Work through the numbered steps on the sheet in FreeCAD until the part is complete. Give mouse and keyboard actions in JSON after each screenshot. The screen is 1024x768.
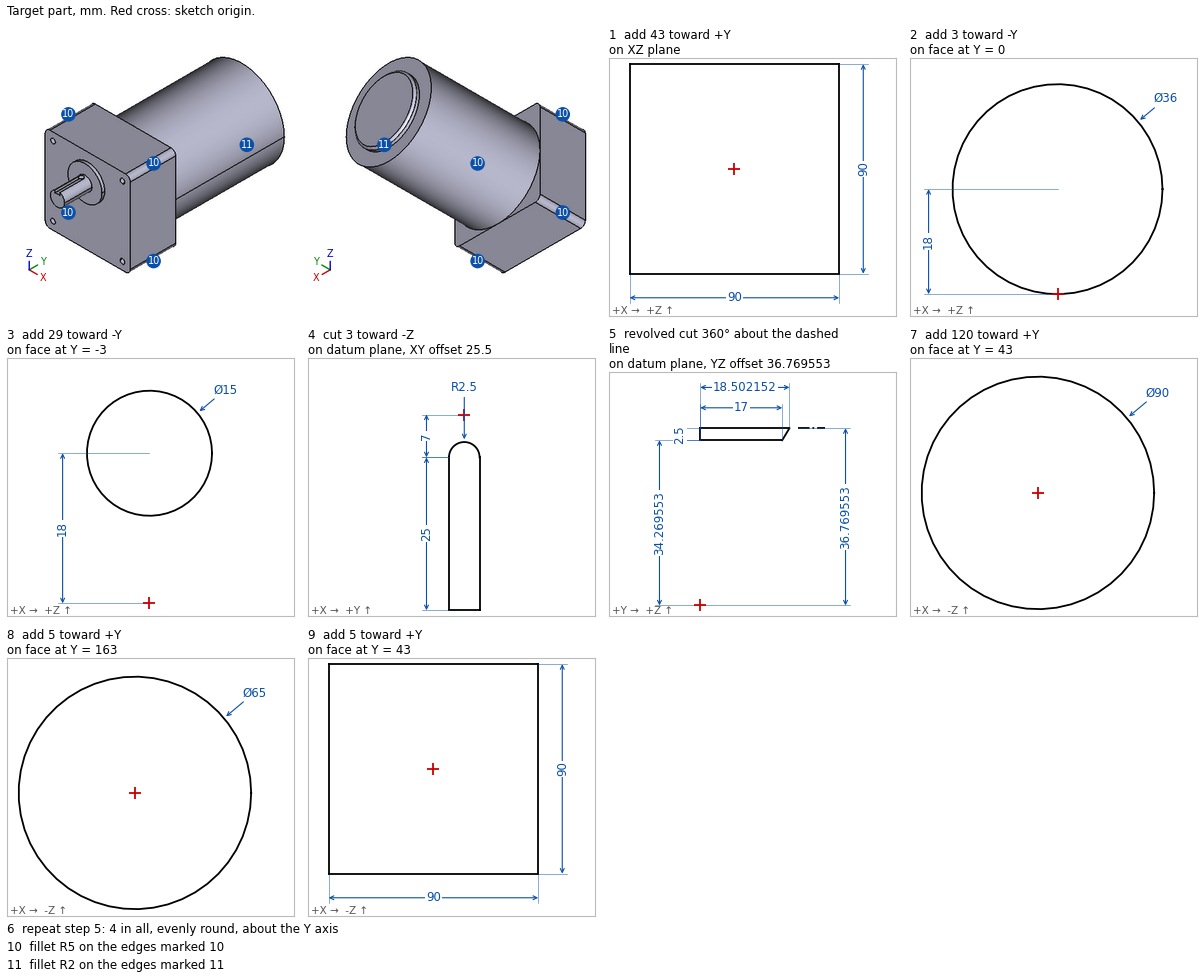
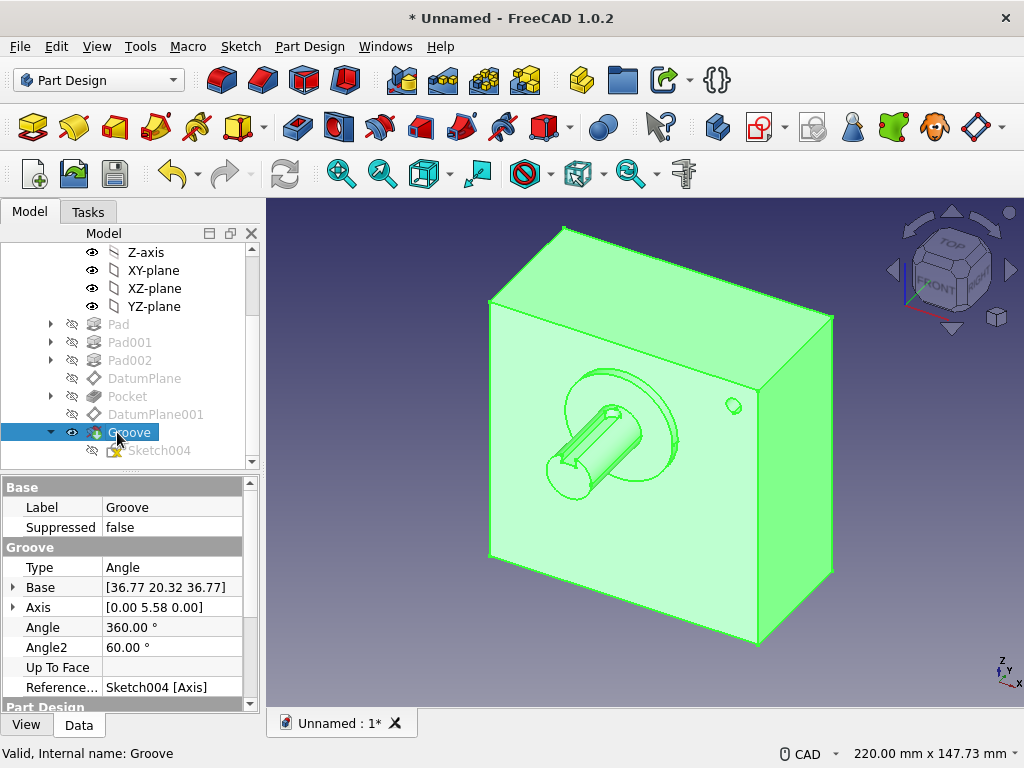
{"action": "left_click", "coordinate": [484, 80]}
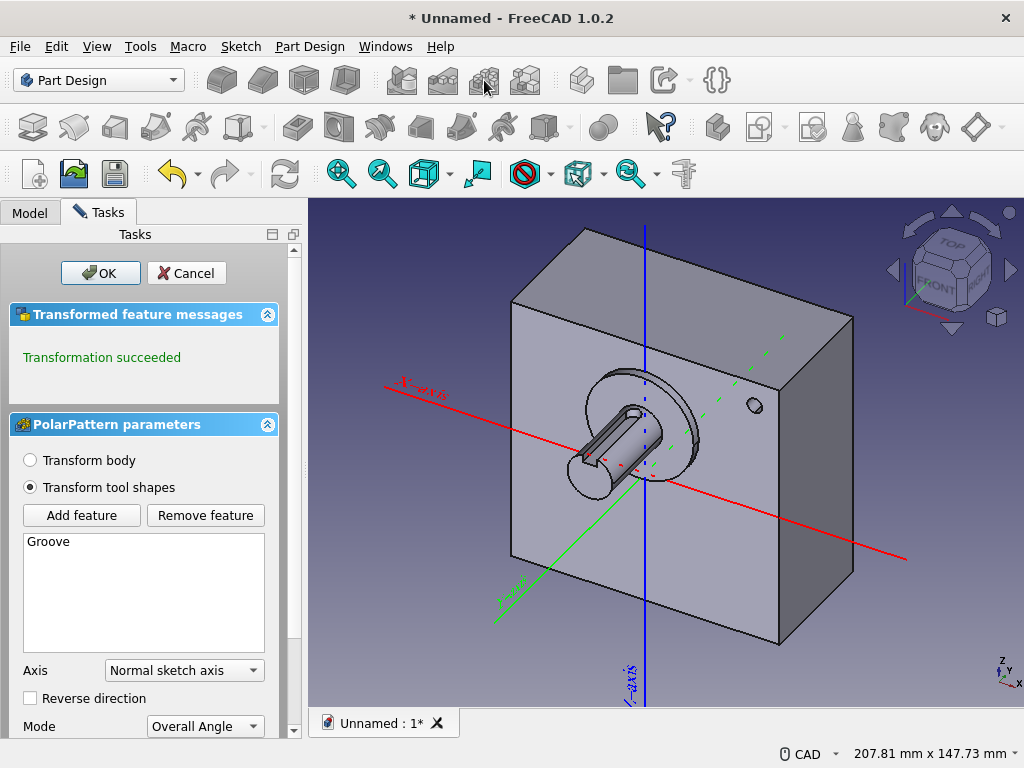
{"action": "left_click", "coordinate": [185, 670]}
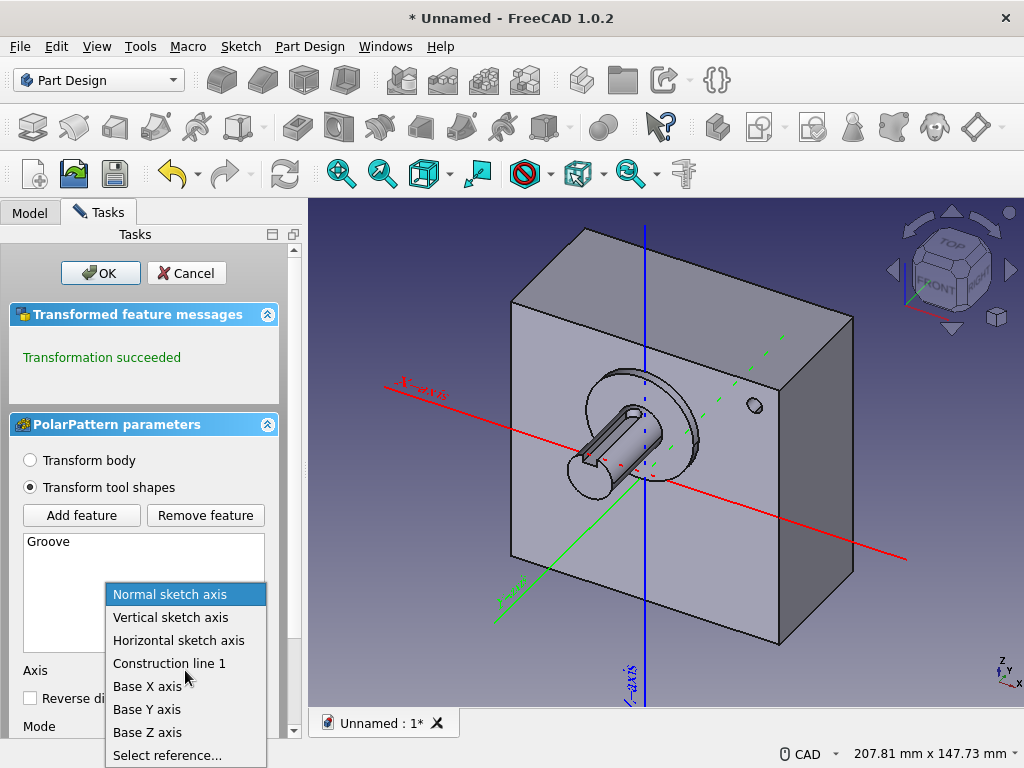
{"action": "left_click", "coordinate": [184, 710]}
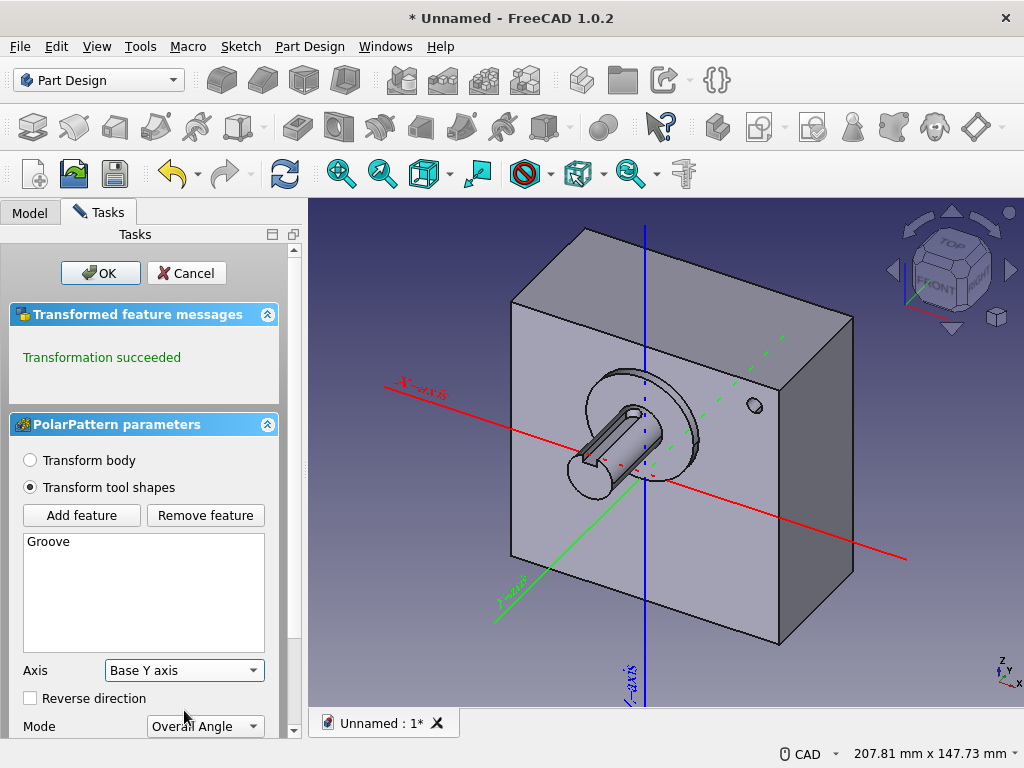
{"action": "scroll", "coordinate": [294, 491], "scroll_direction": "down", "scroll_amount": 3}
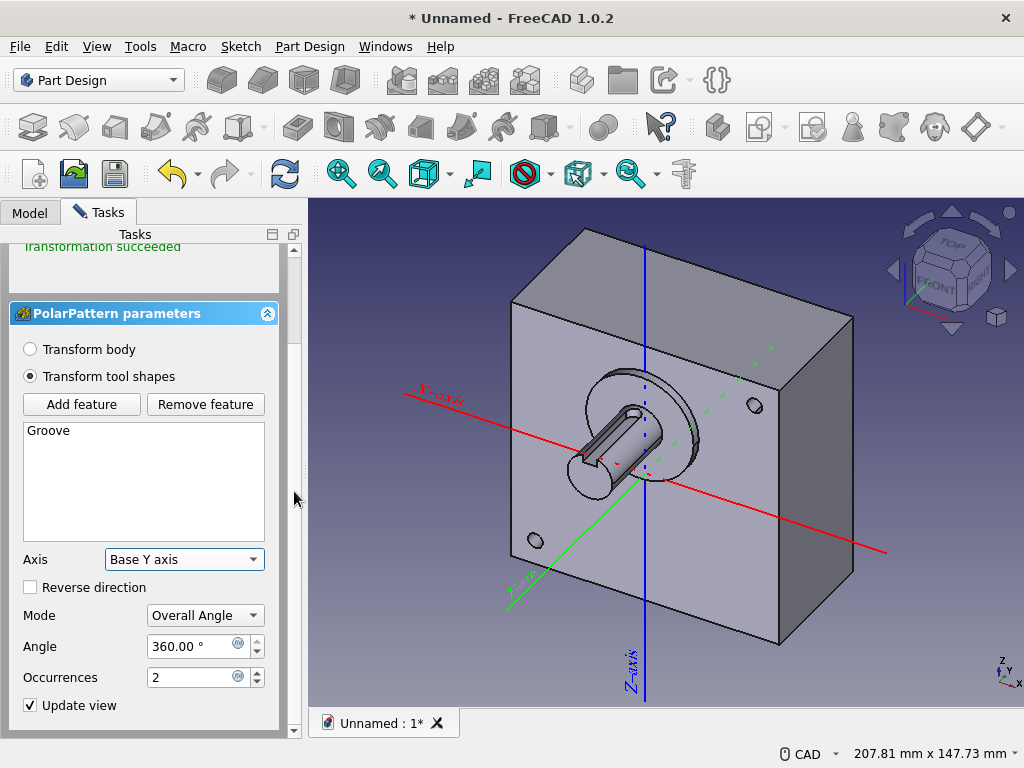
{"action": "triple_click", "coordinate": [199, 678]}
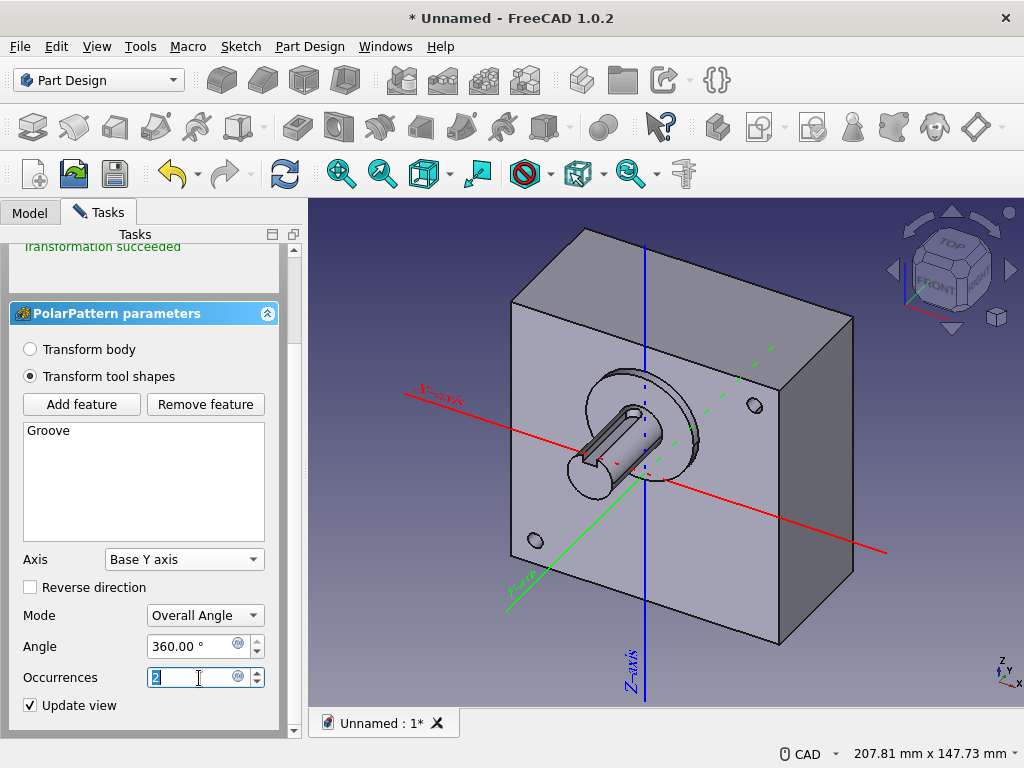
{"action": "type", "text": "4"}
{"action": "key", "text": "Tab"}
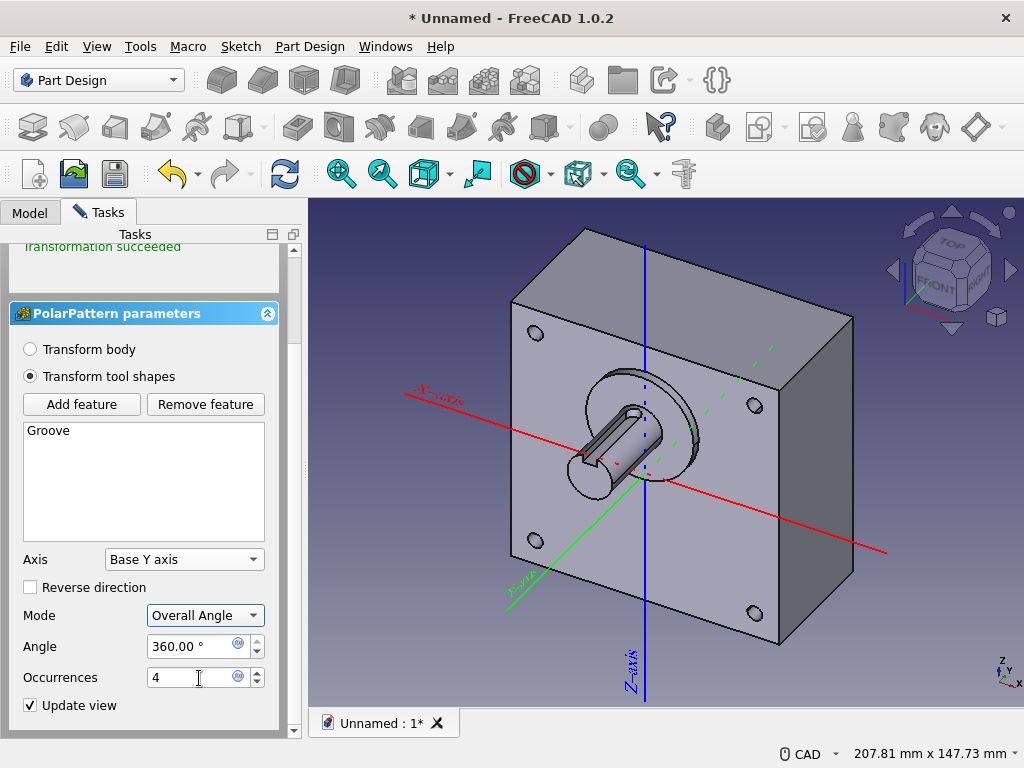
{"action": "scroll", "coordinate": [294, 491], "scroll_direction": "up", "scroll_amount": 3}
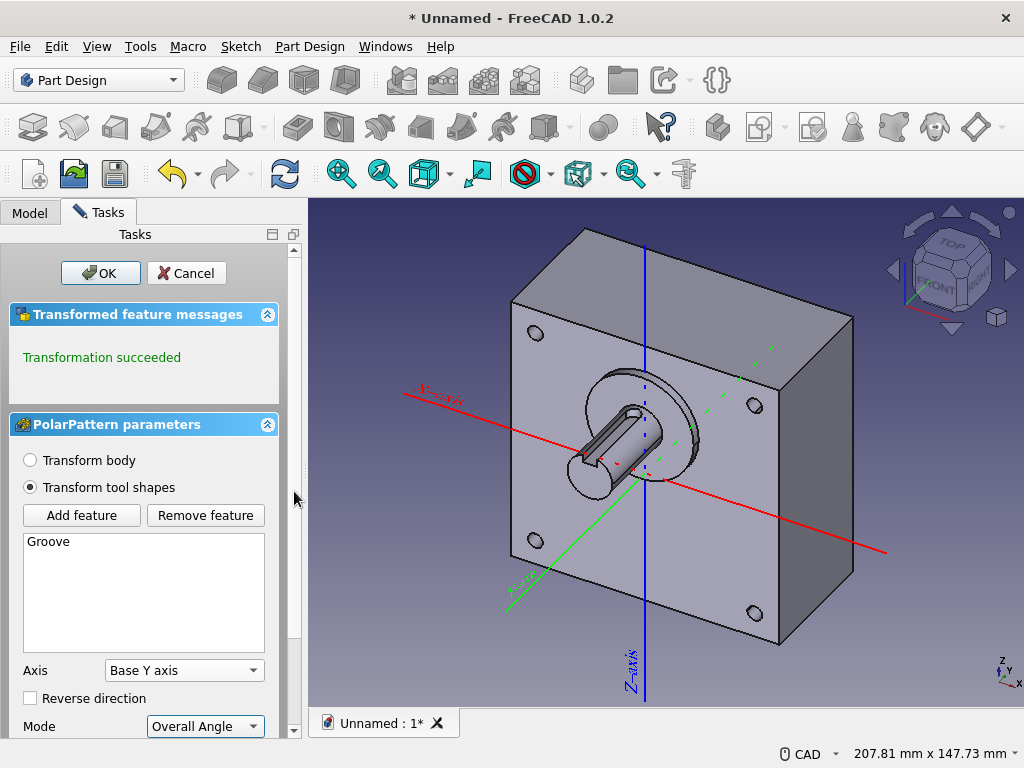
{"action": "left_click", "coordinate": [101, 273]}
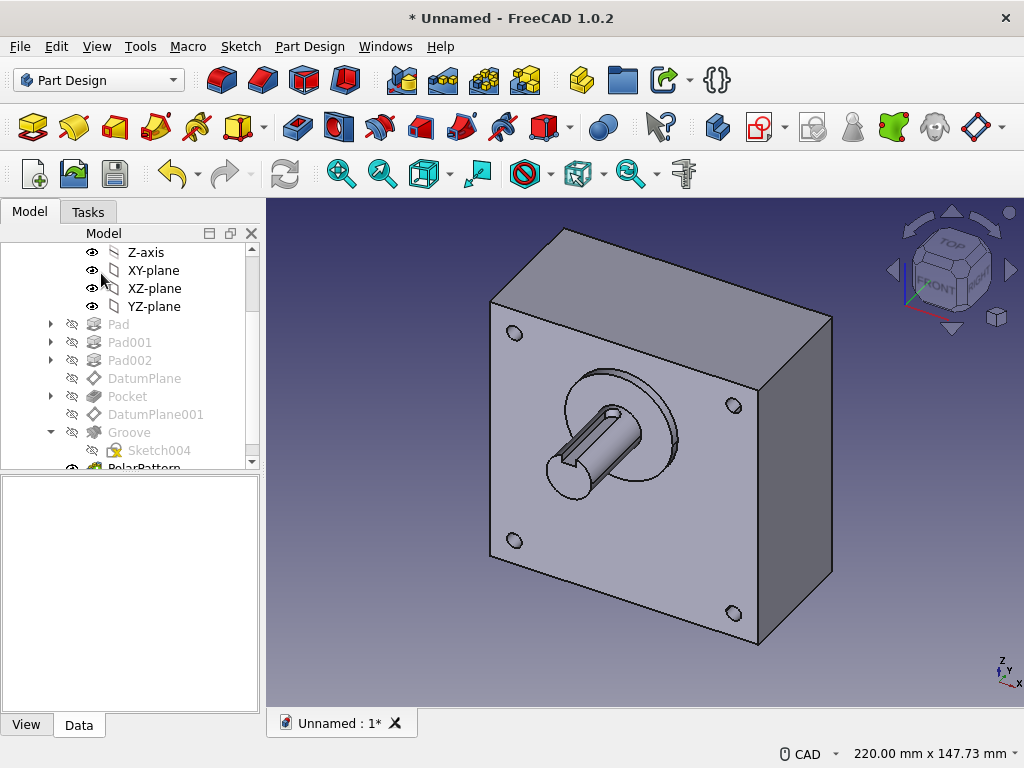
{"action": "key", "text": "4"}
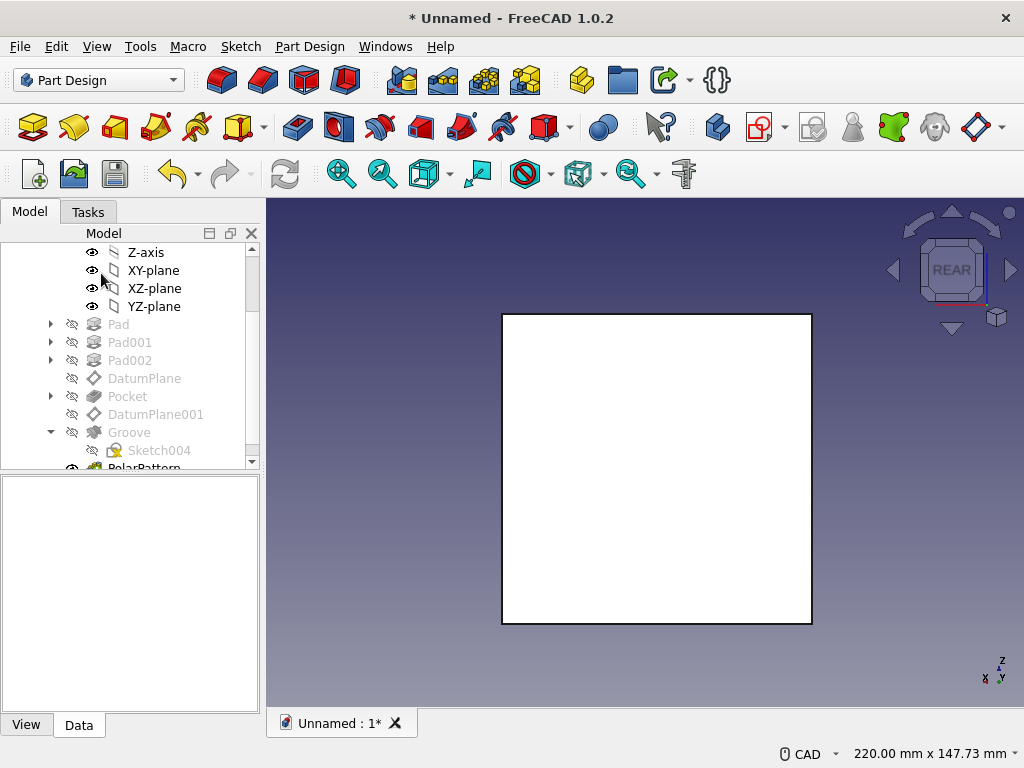
{"action": "left_click", "coordinate": [657, 468]}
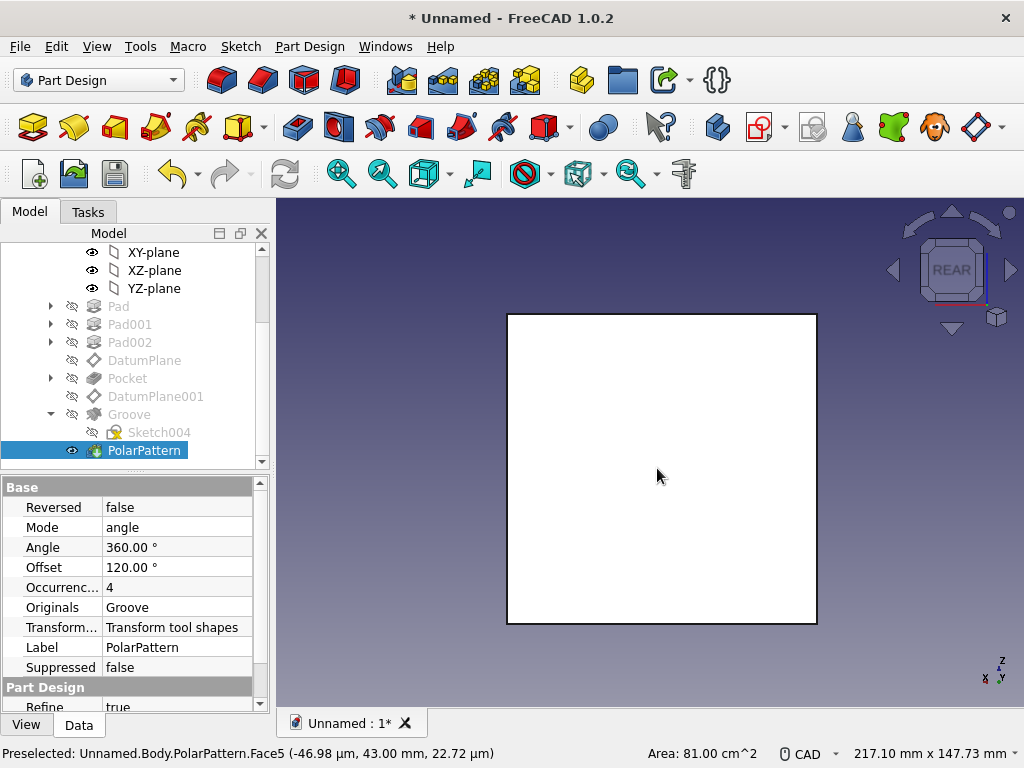
{"action": "left_click", "coordinate": [758, 128]}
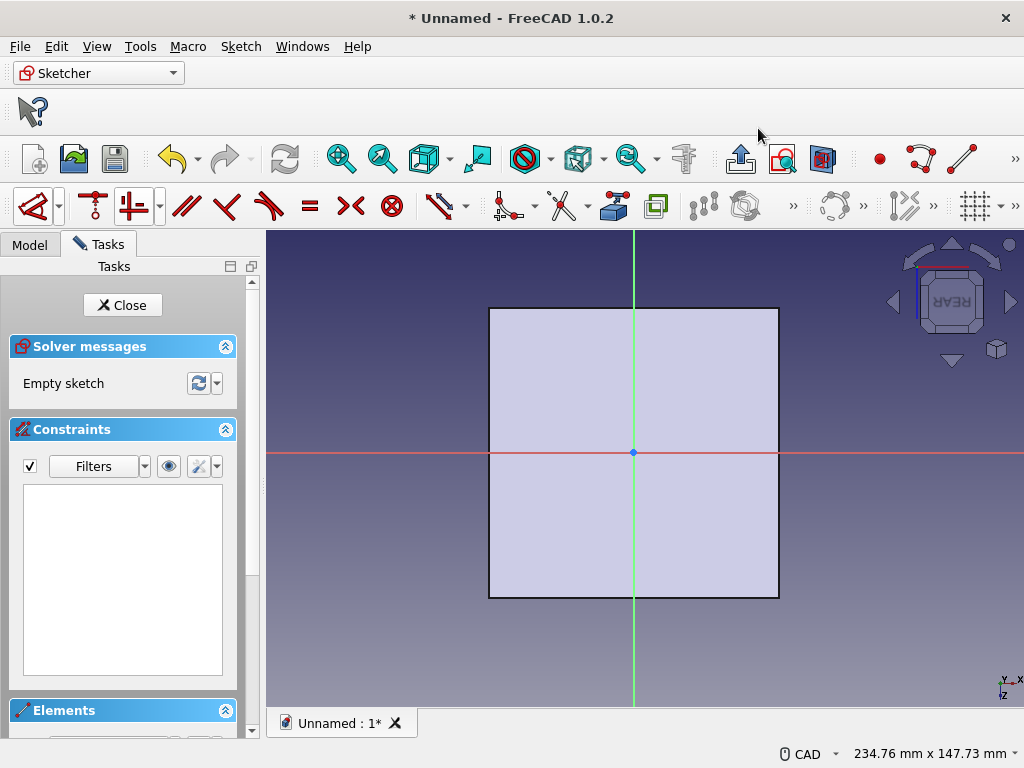
{"action": "key", "text": "g c"}